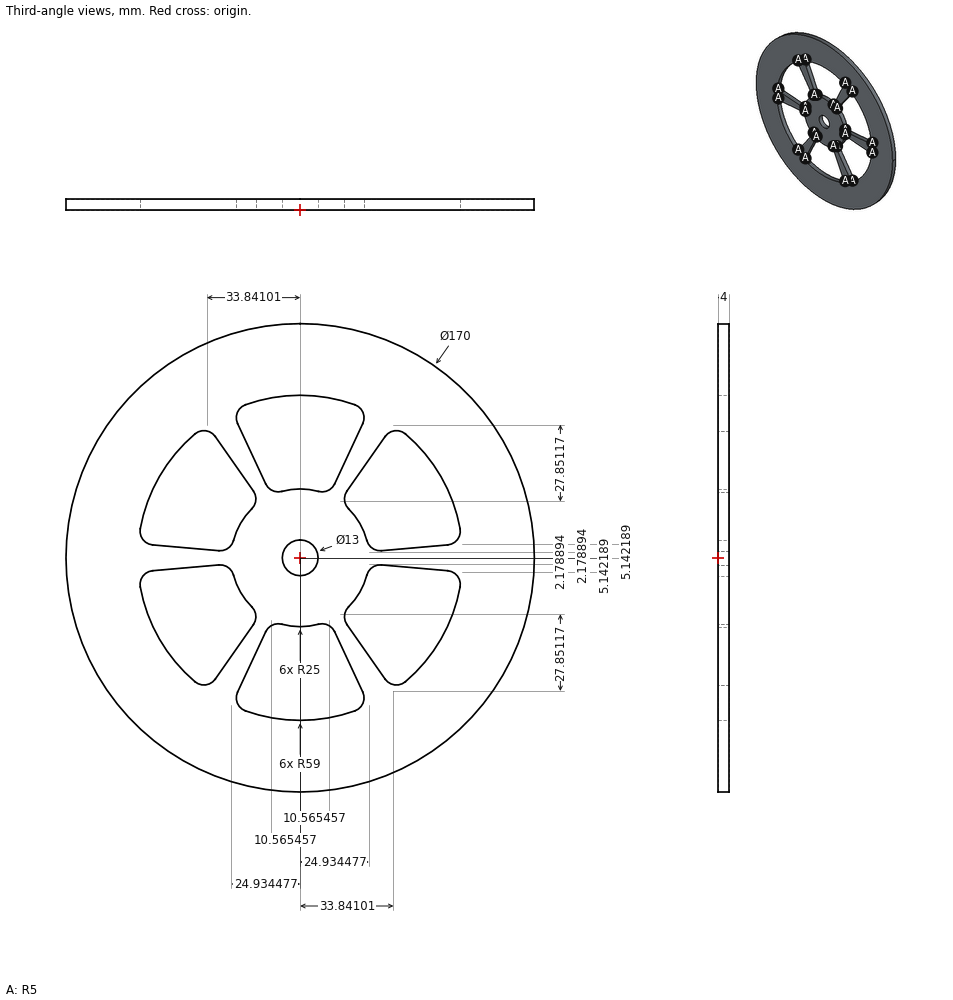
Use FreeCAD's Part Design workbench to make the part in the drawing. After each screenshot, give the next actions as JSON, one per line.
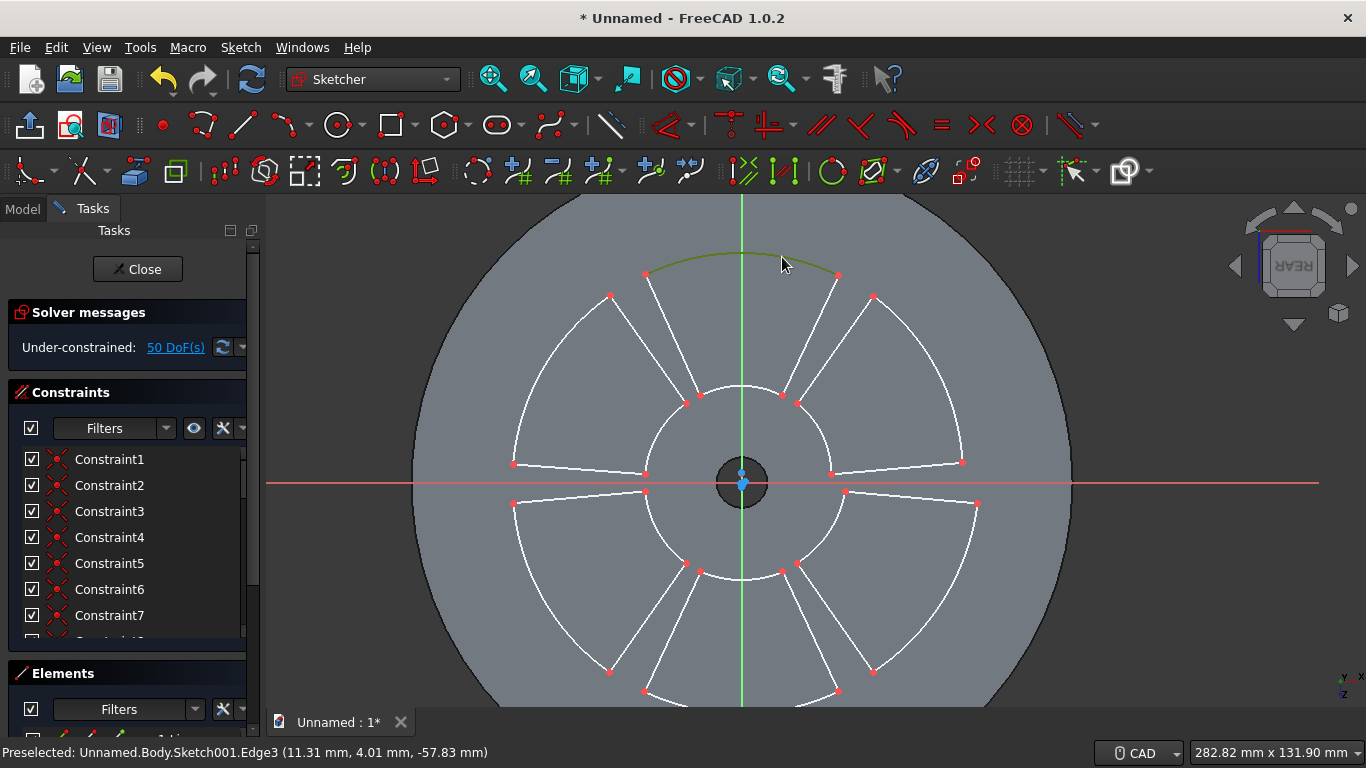
{"action": "left_click", "coordinate": [725, 579]}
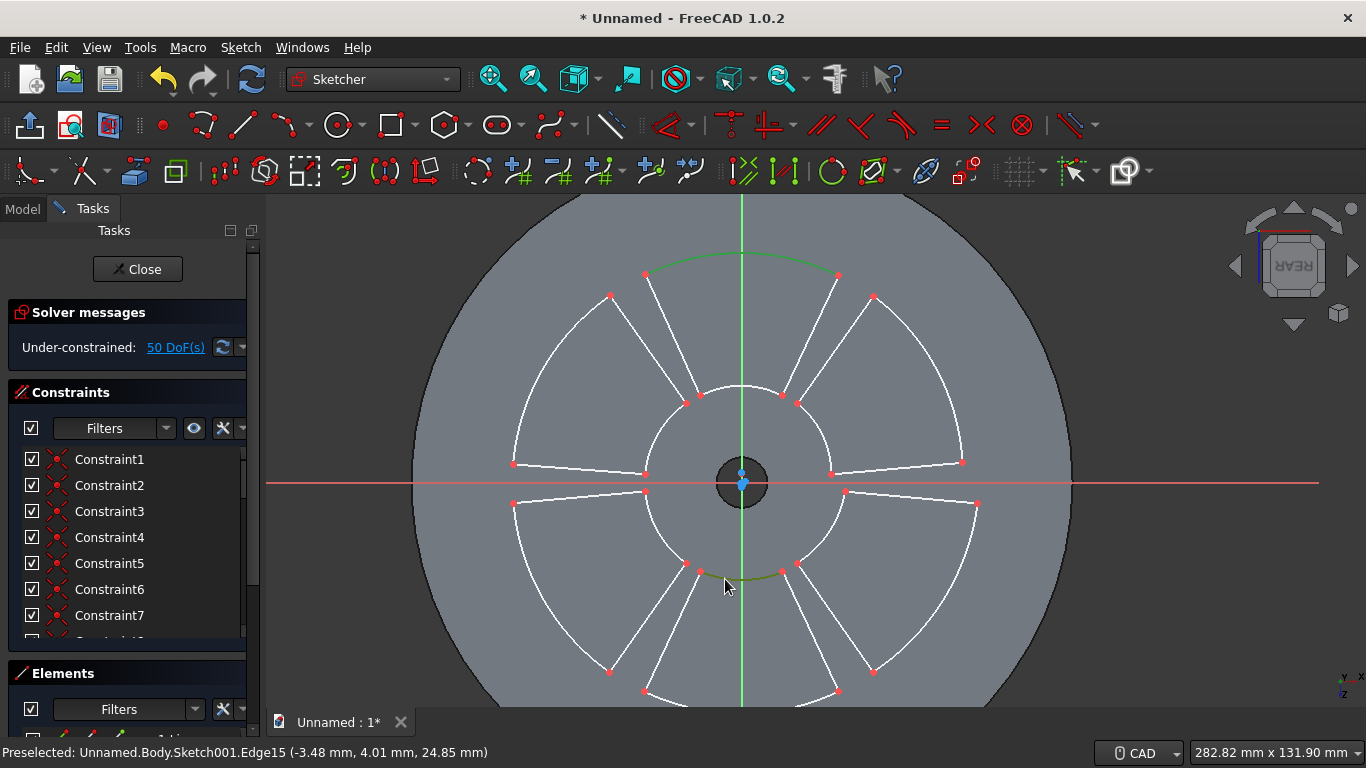
{"action": "left_click", "coordinate": [730, 126]}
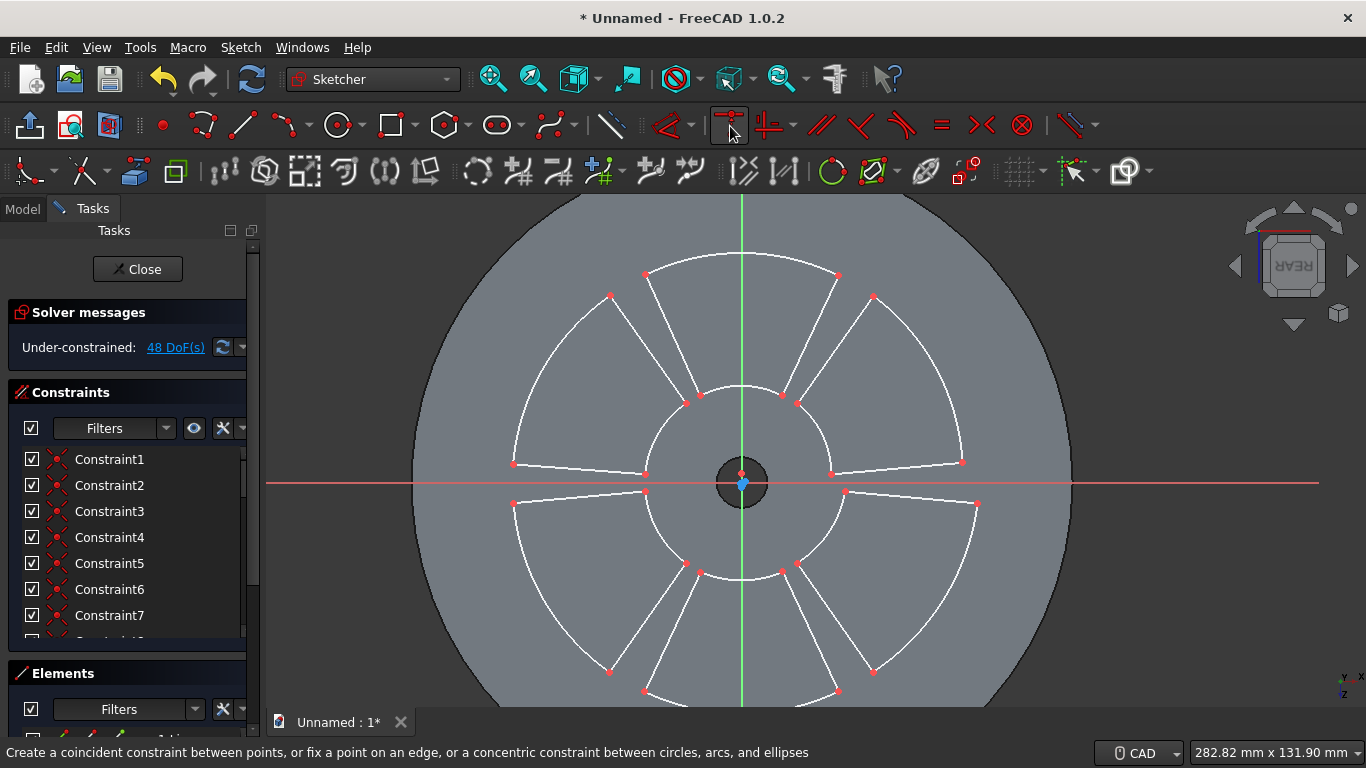
{"action": "left_click", "coordinate": [782, 257]}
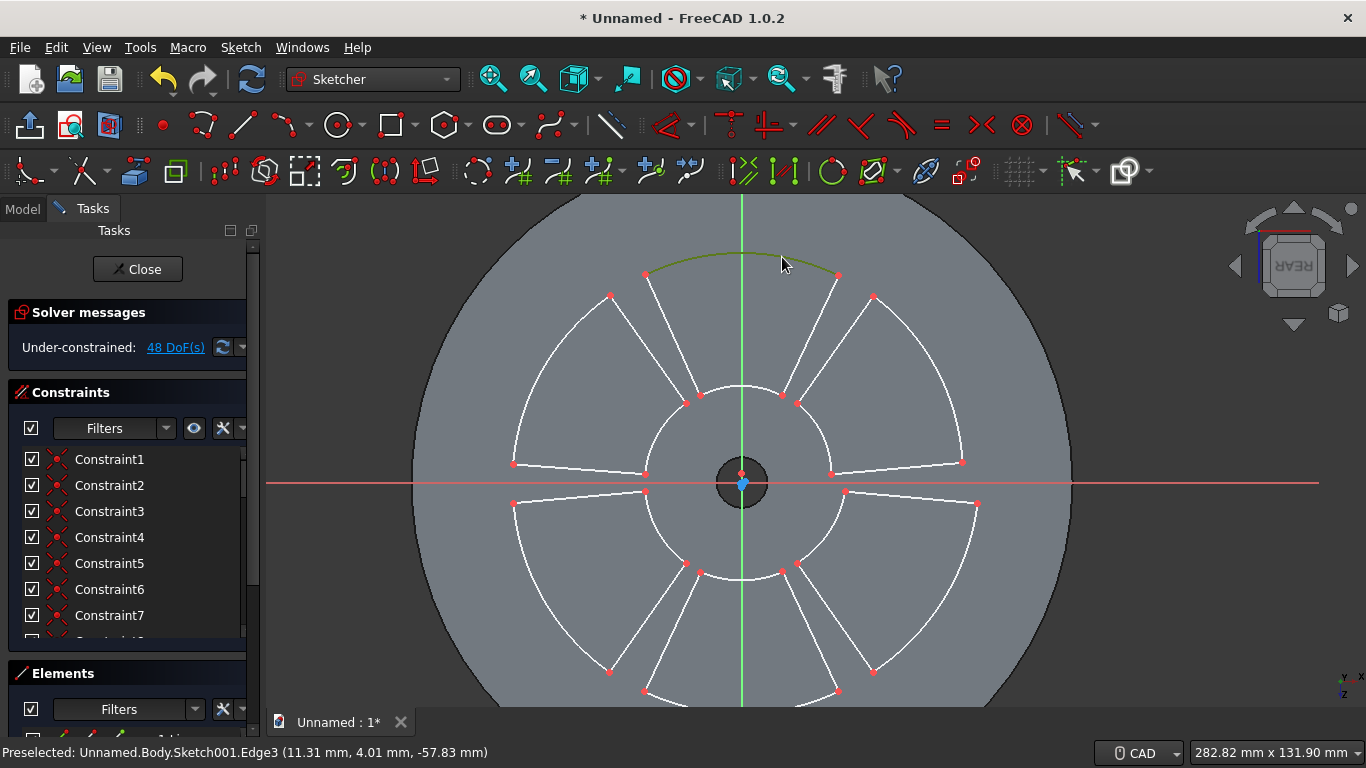
{"action": "scroll", "coordinate": [759, 385], "scroll_direction": "down", "scroll_amount": 2}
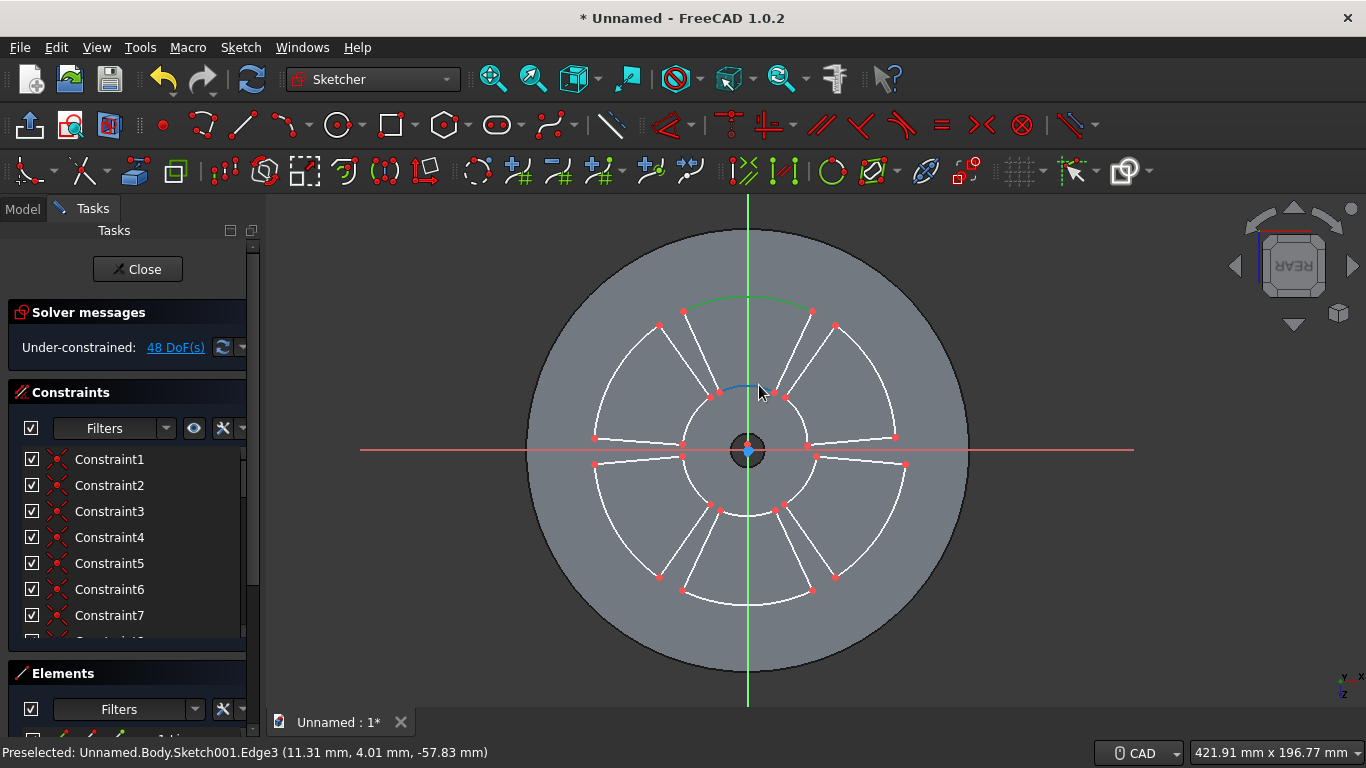
{"action": "left_click", "coordinate": [721, 603]}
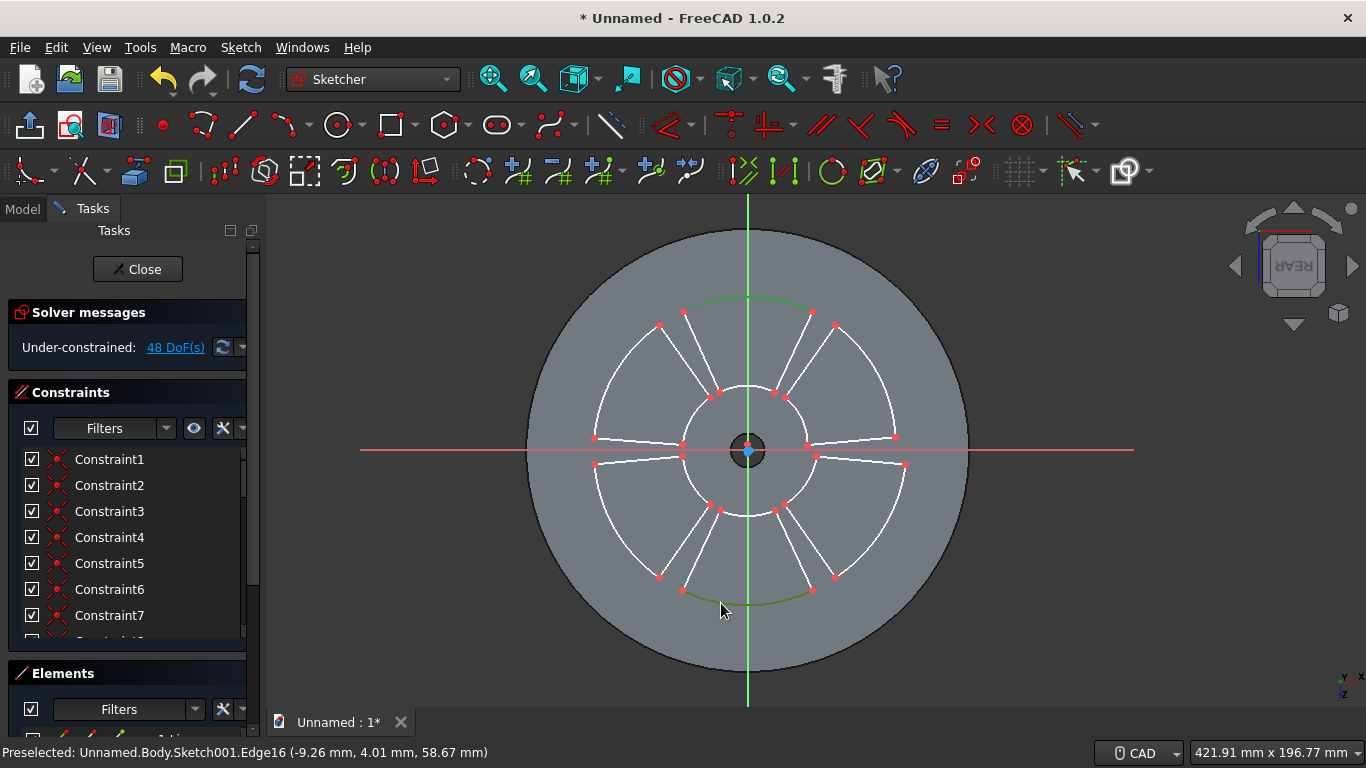
{"action": "left_click", "coordinate": [730, 126]}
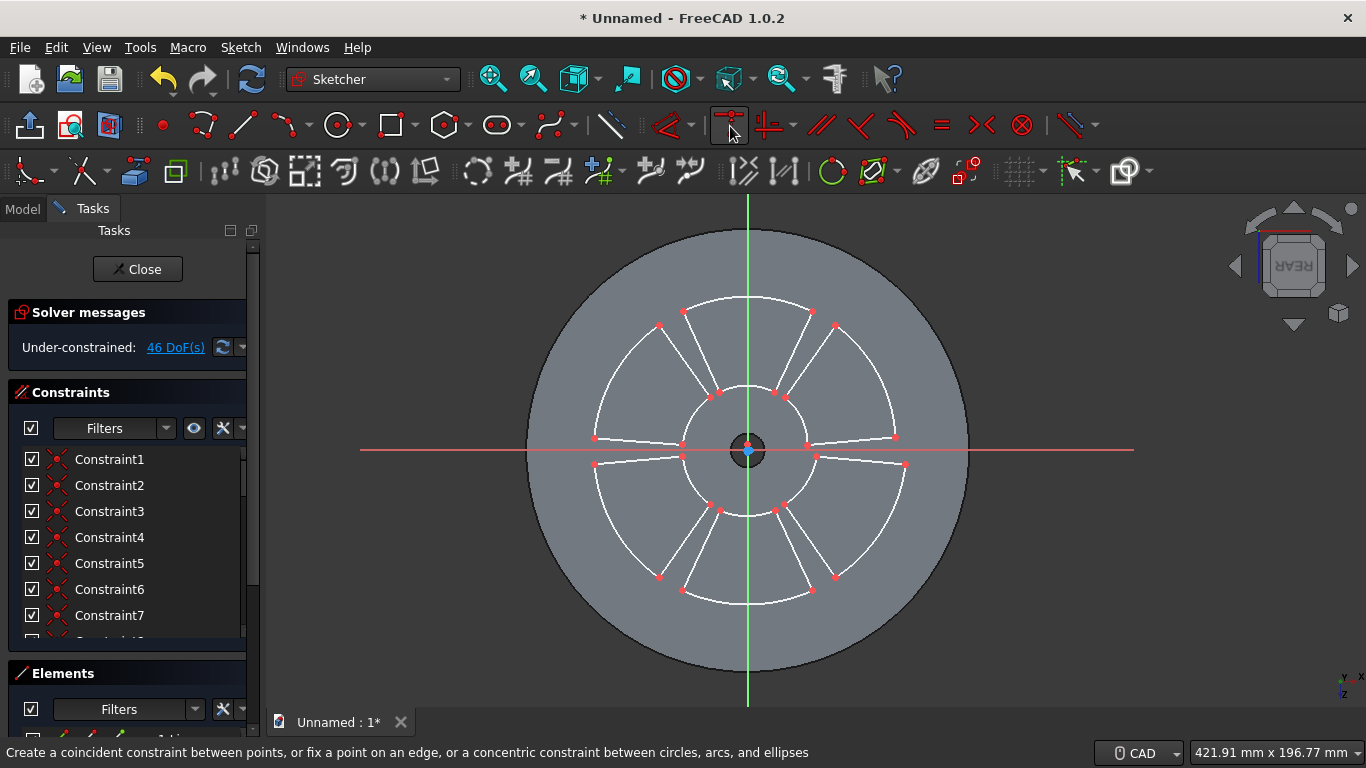
{"action": "left_click", "coordinate": [775, 299]}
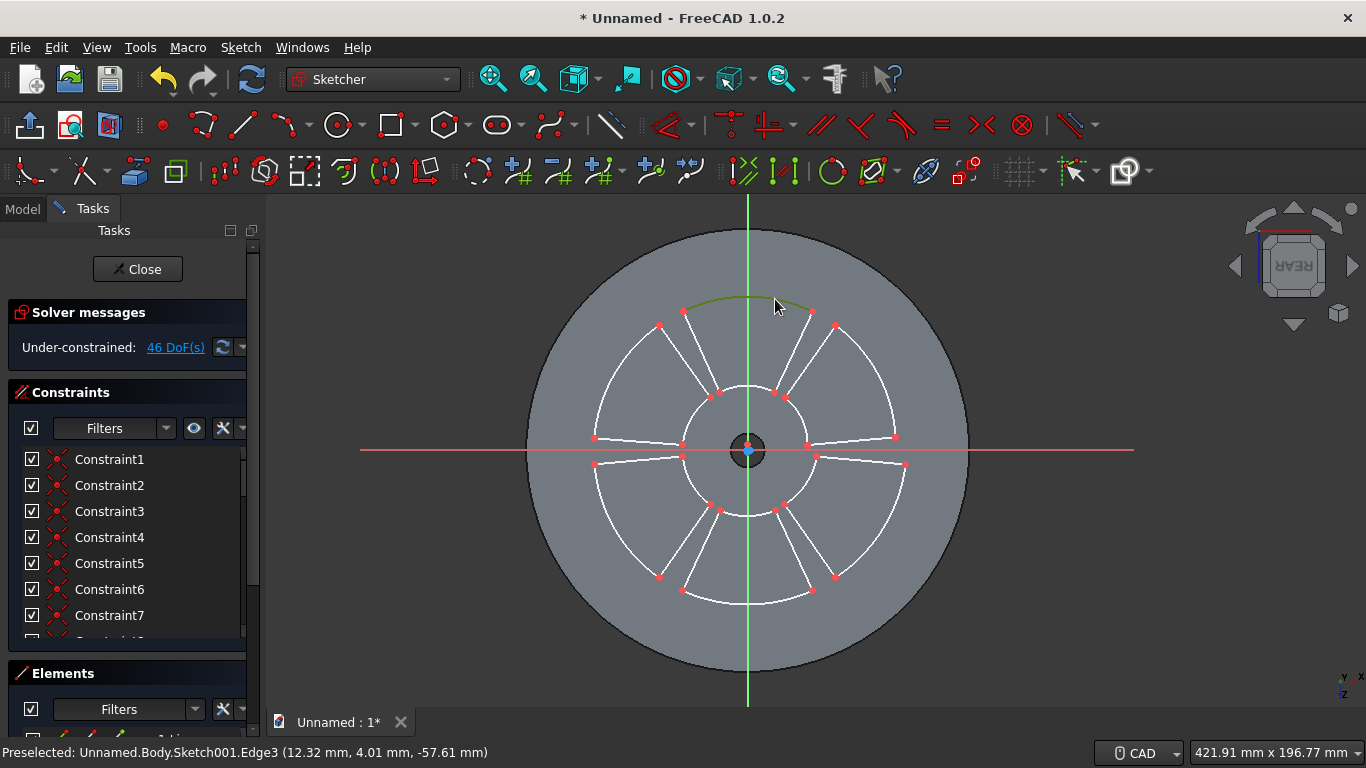
{"action": "left_click", "coordinate": [687, 473]}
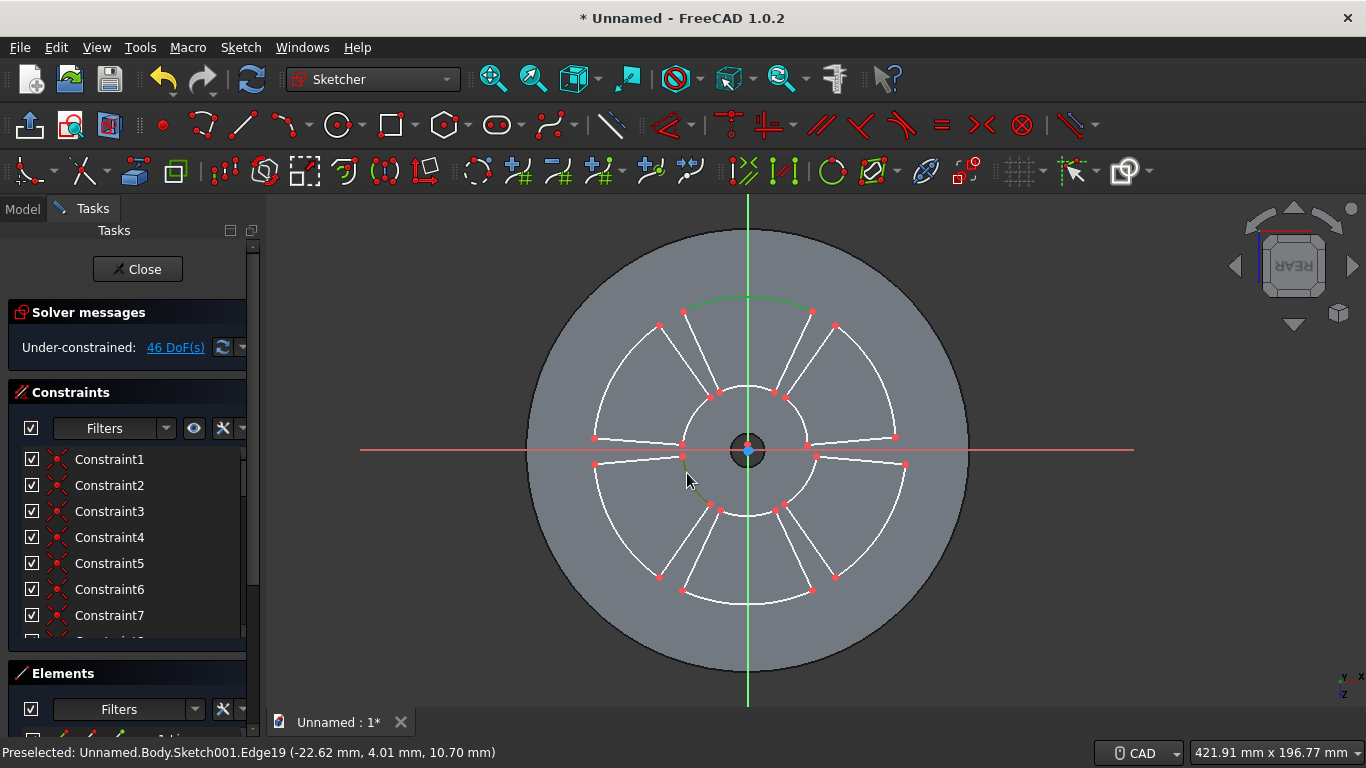
{"action": "left_click", "coordinate": [730, 126]}